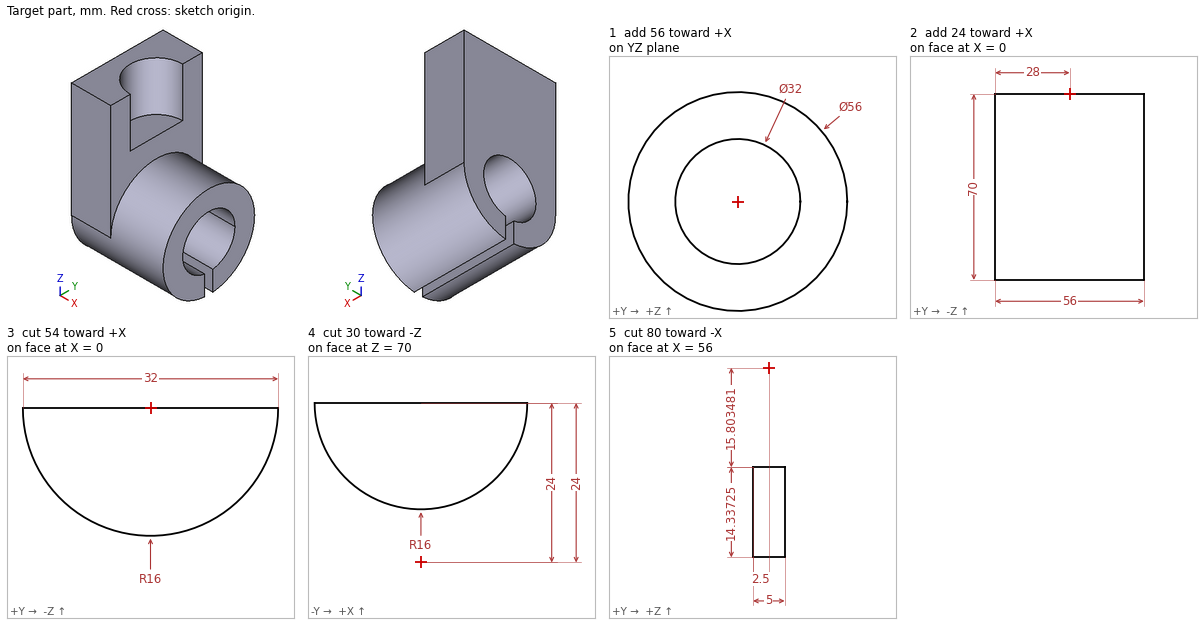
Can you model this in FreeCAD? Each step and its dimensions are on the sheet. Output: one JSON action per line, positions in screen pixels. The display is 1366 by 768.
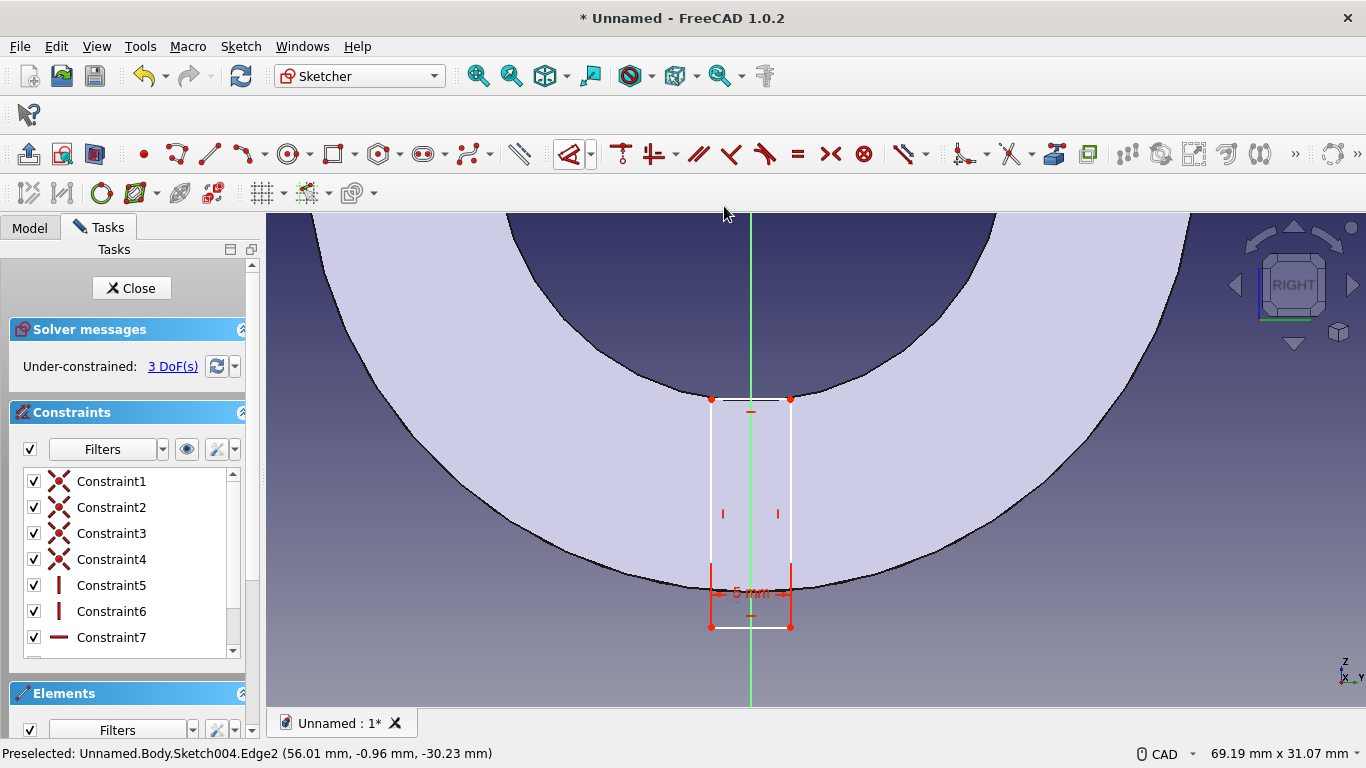
{"action": "left_click", "coordinate": [711, 399]}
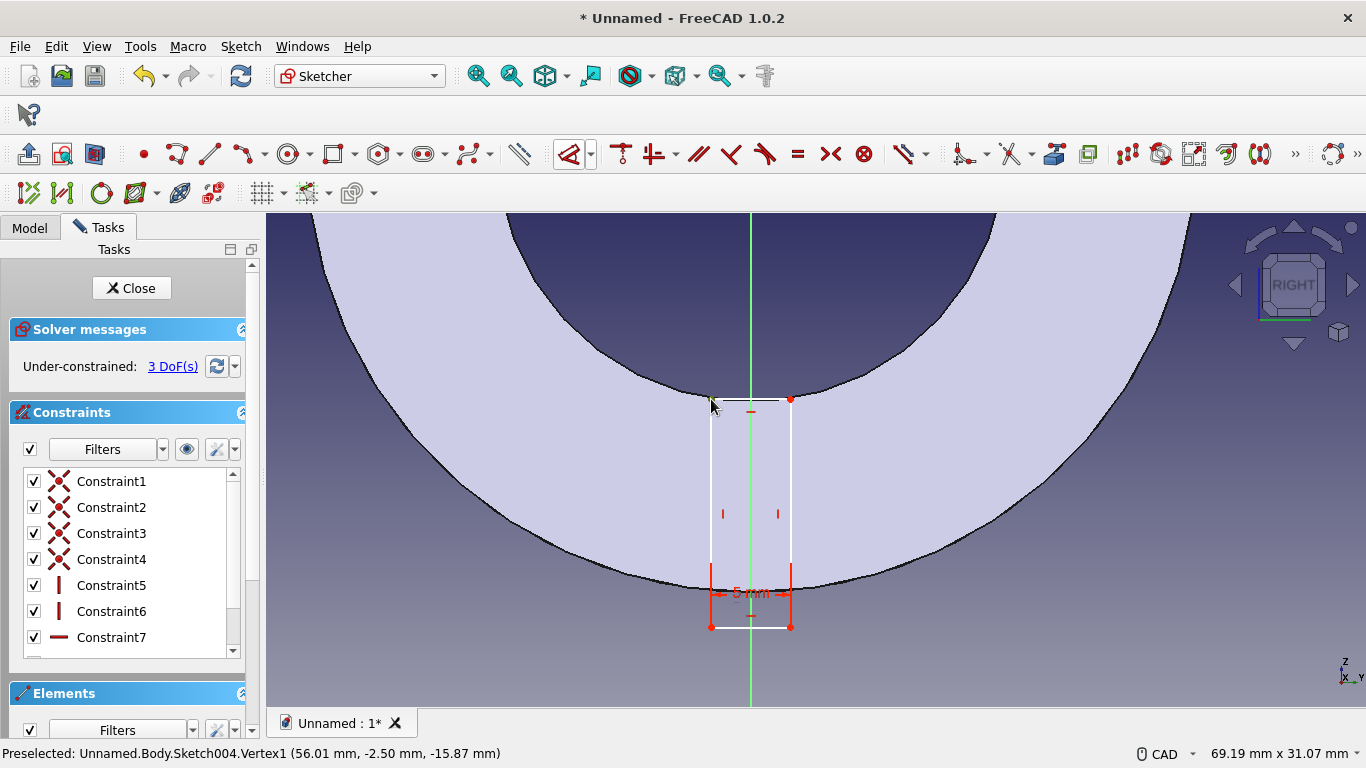
{"action": "left_click", "coordinate": [590, 154]}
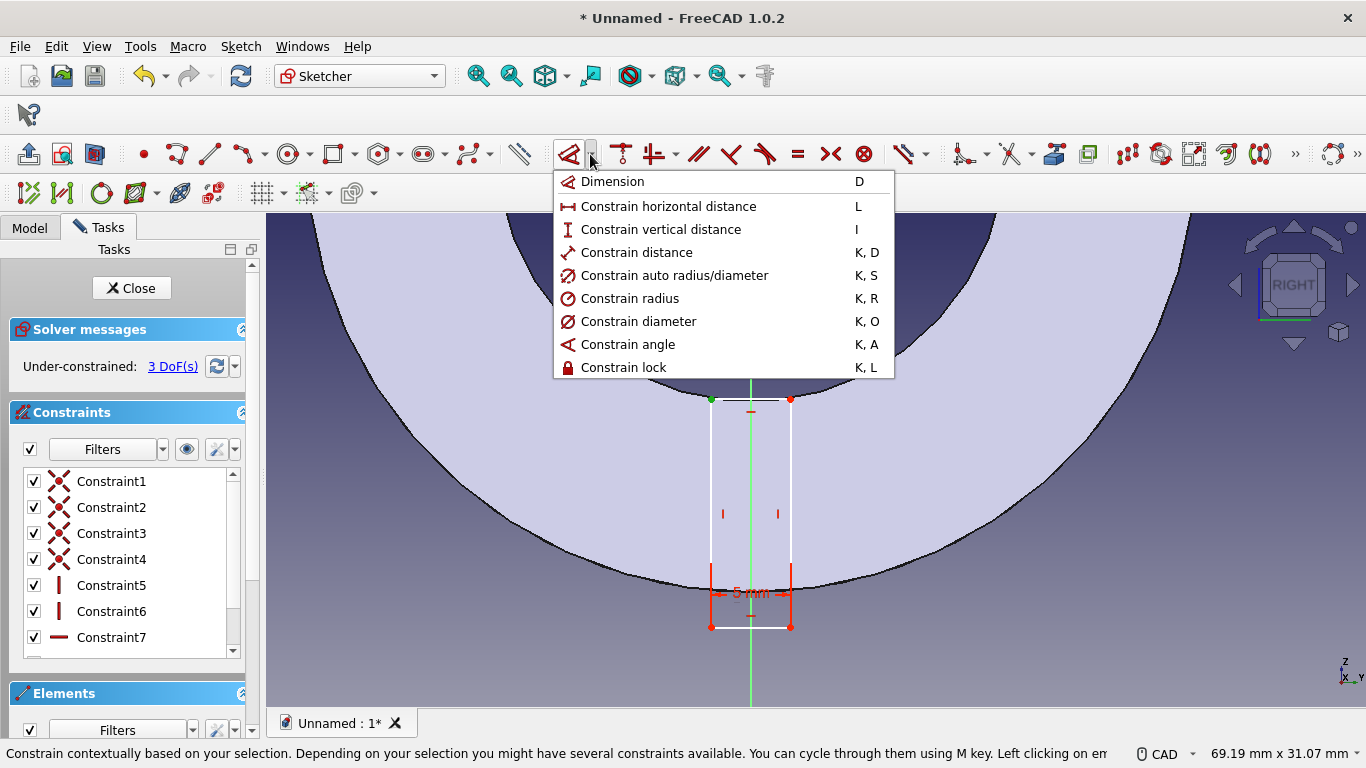
{"action": "left_click", "coordinate": [724, 206]}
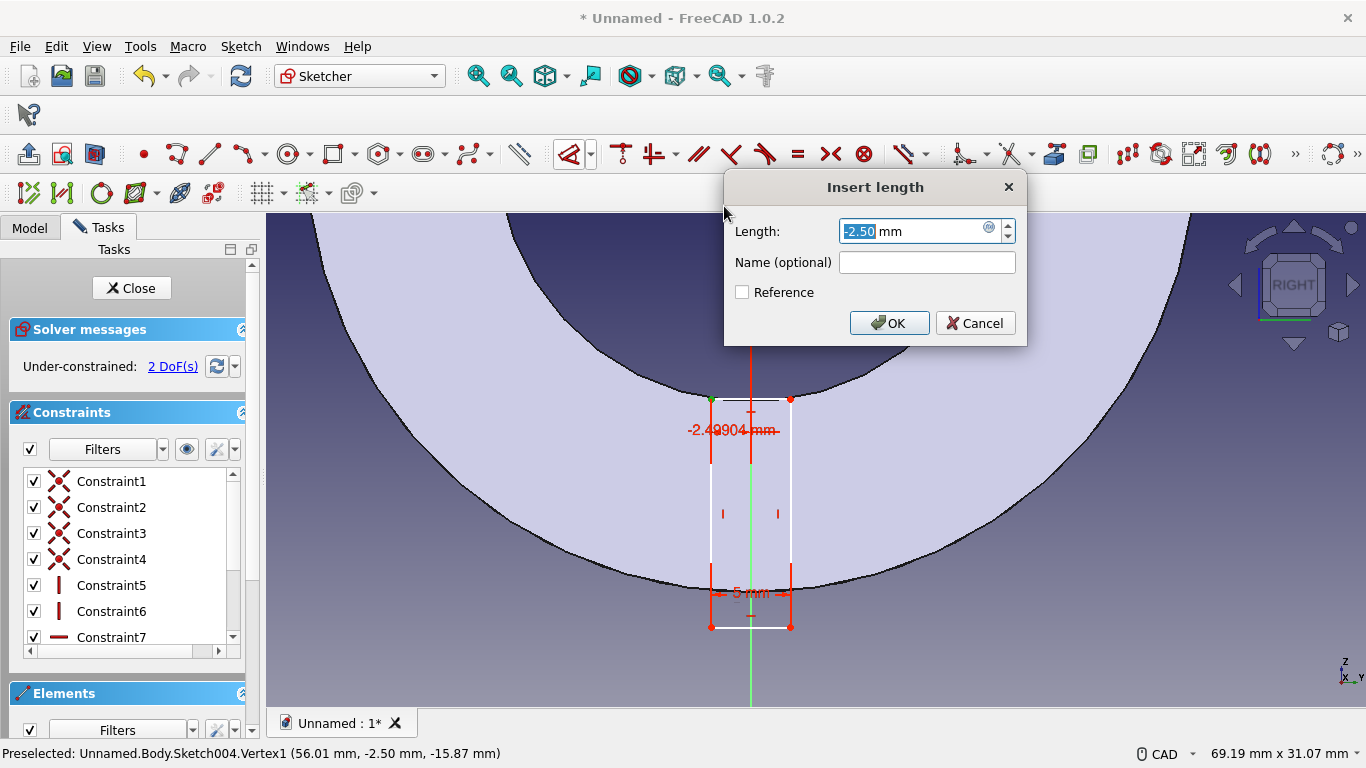
{"action": "type", "text": "-2.5"}
{"action": "key", "text": "Return"}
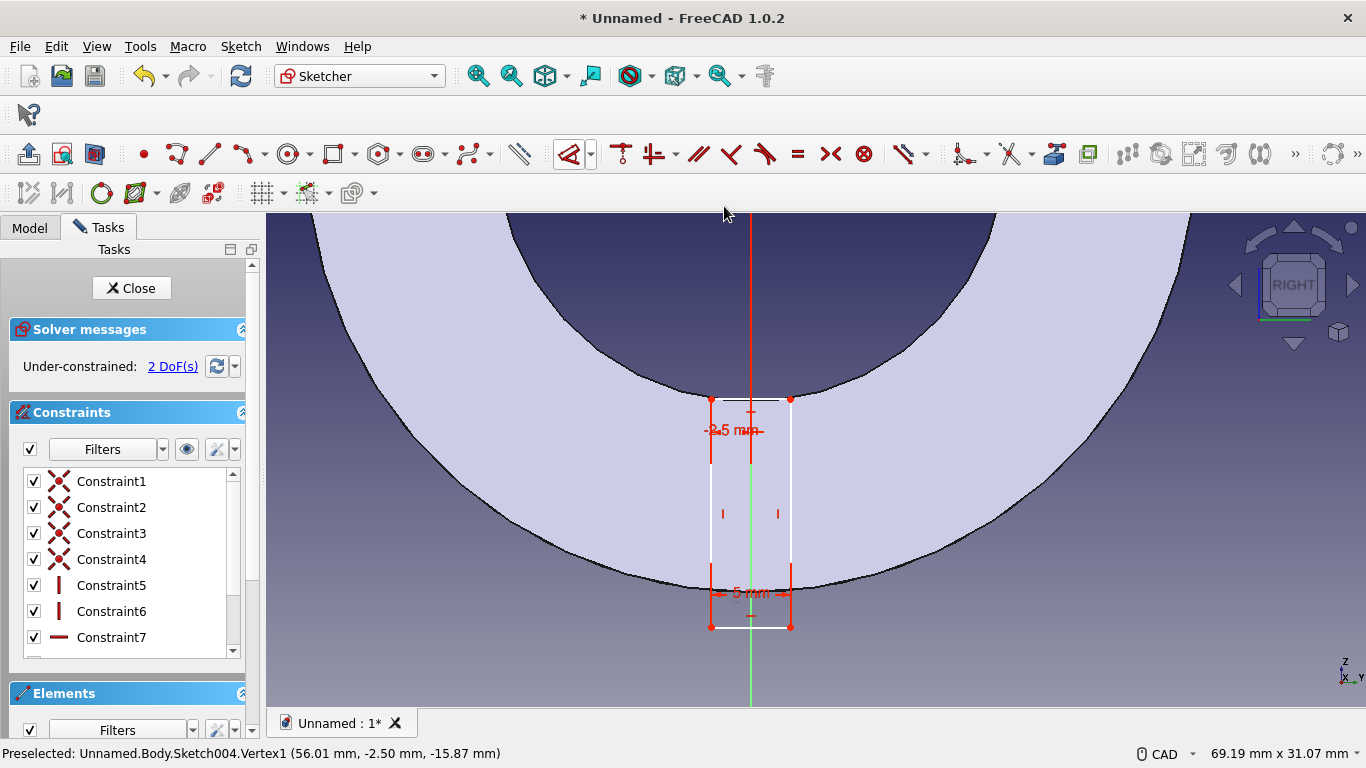
{"action": "left_click", "coordinate": [711, 468]}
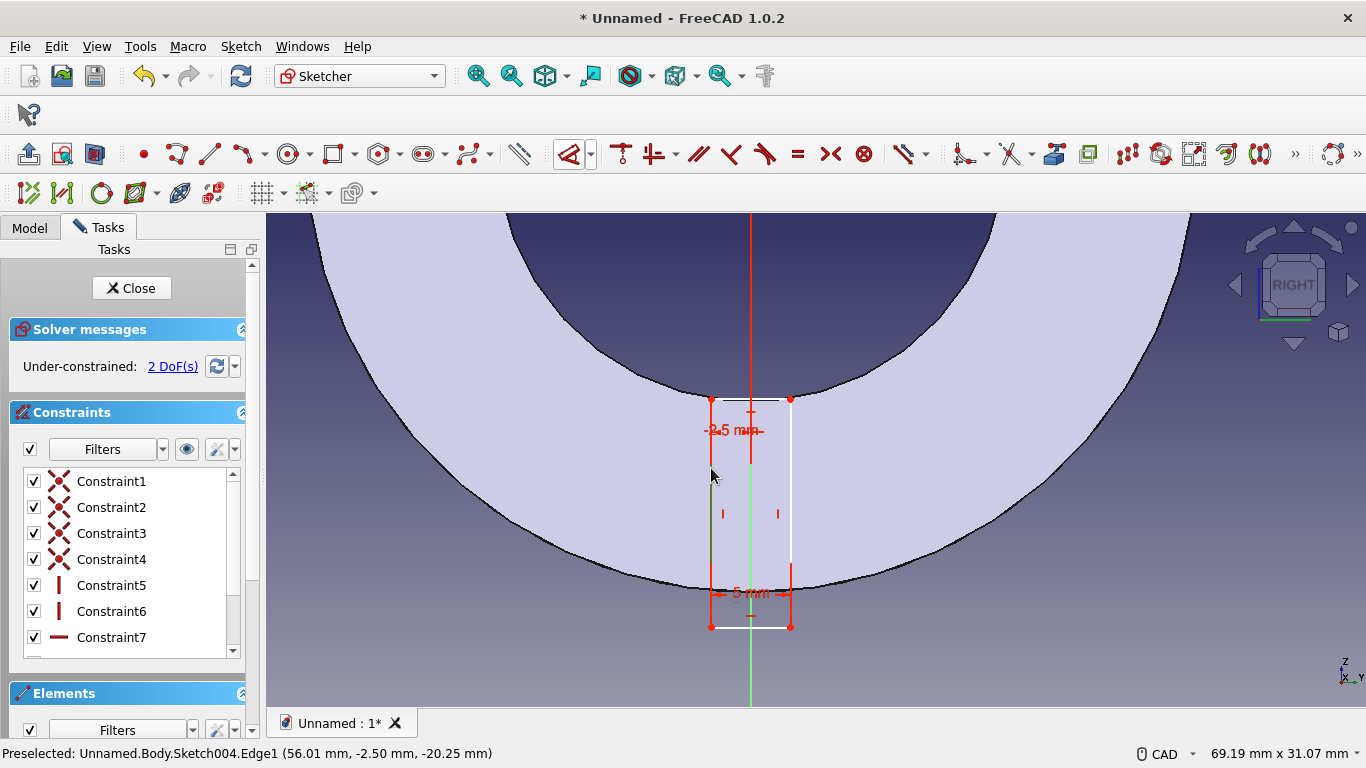
{"action": "key", "text": "i"}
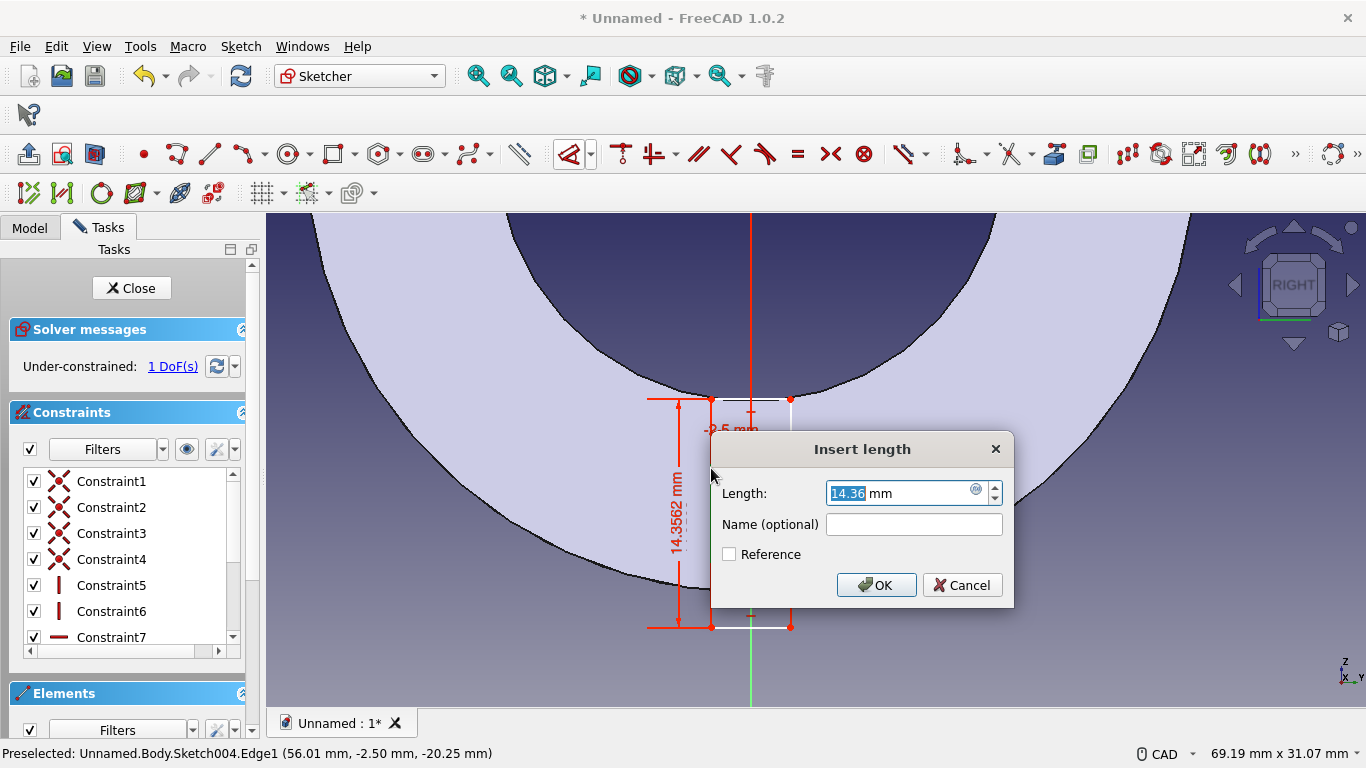
{"action": "type", "text": "14.33725"}
{"action": "key", "text": "Return"}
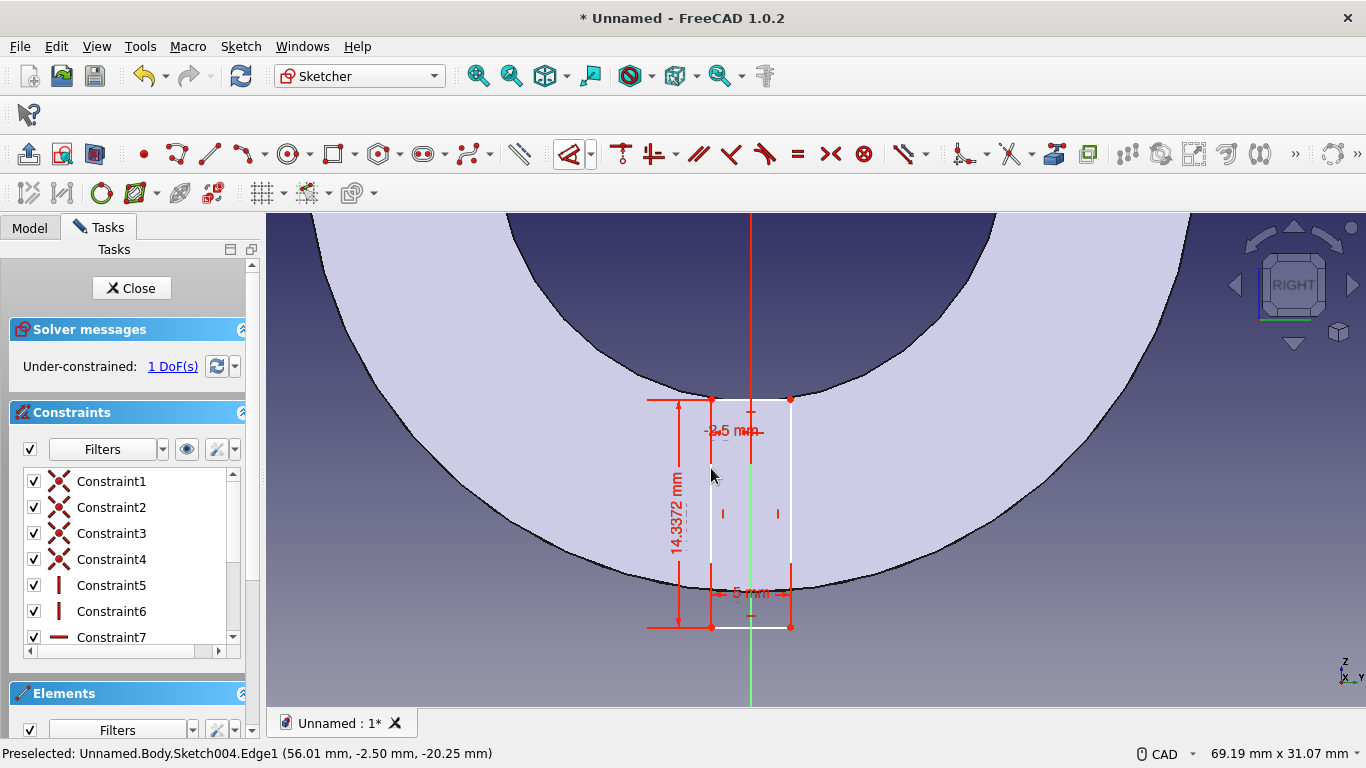
{"action": "left_click", "coordinate": [711, 400]}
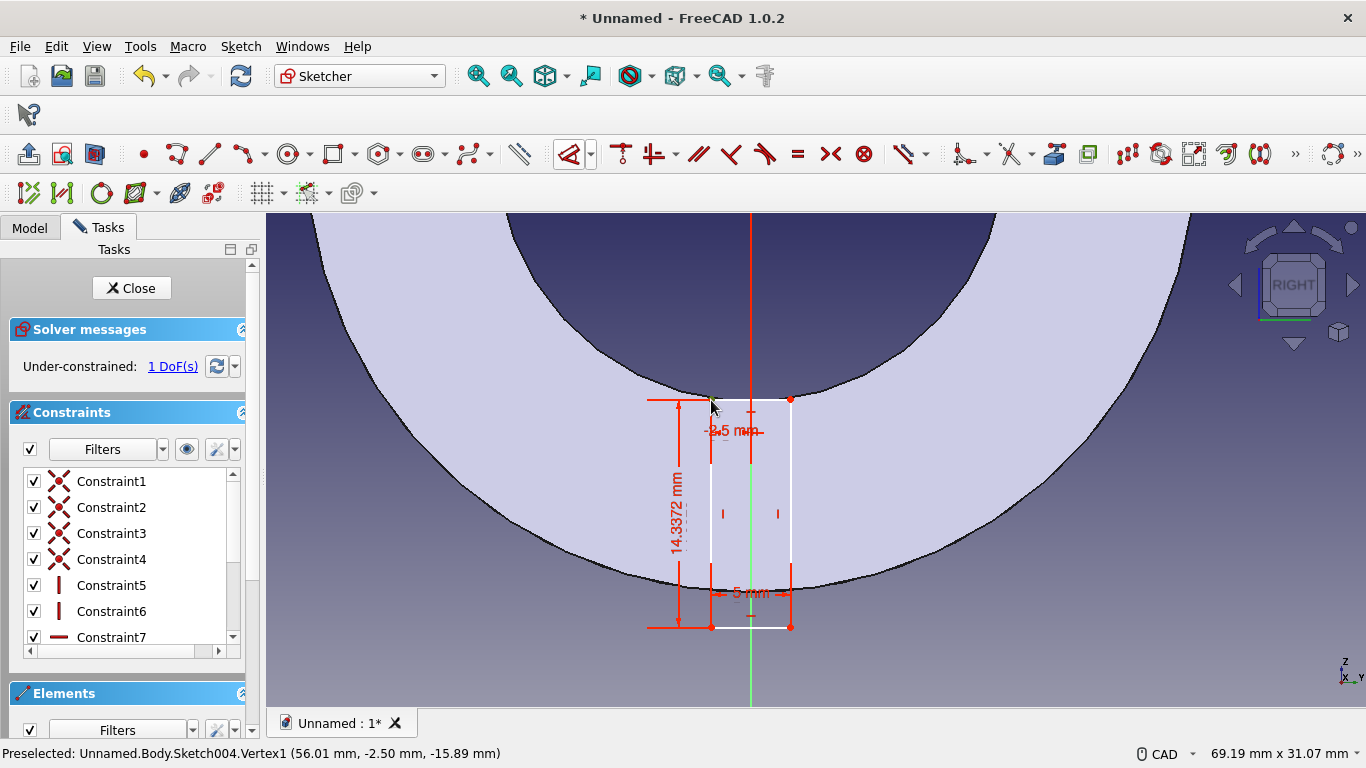
{"action": "left_click", "coordinate": [590, 154]}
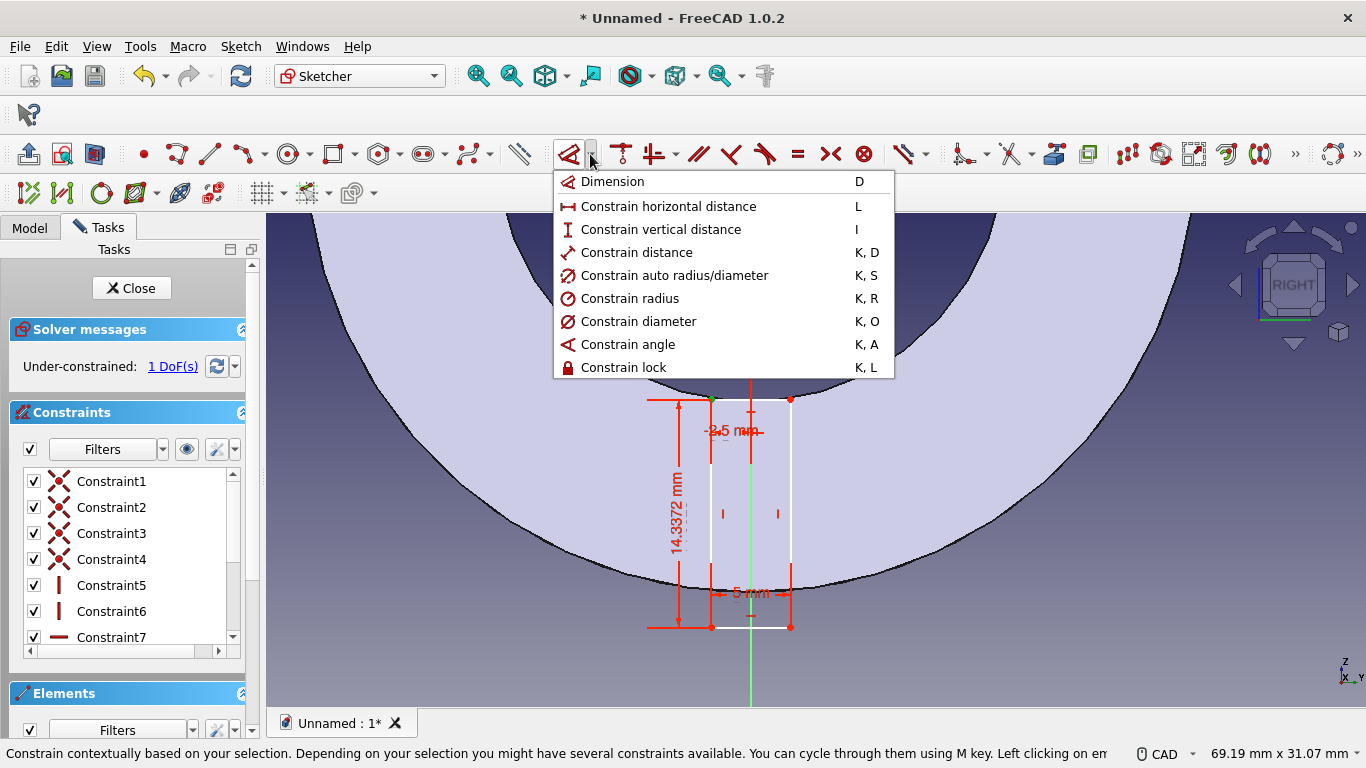
{"action": "left_click", "coordinate": [724, 230]}